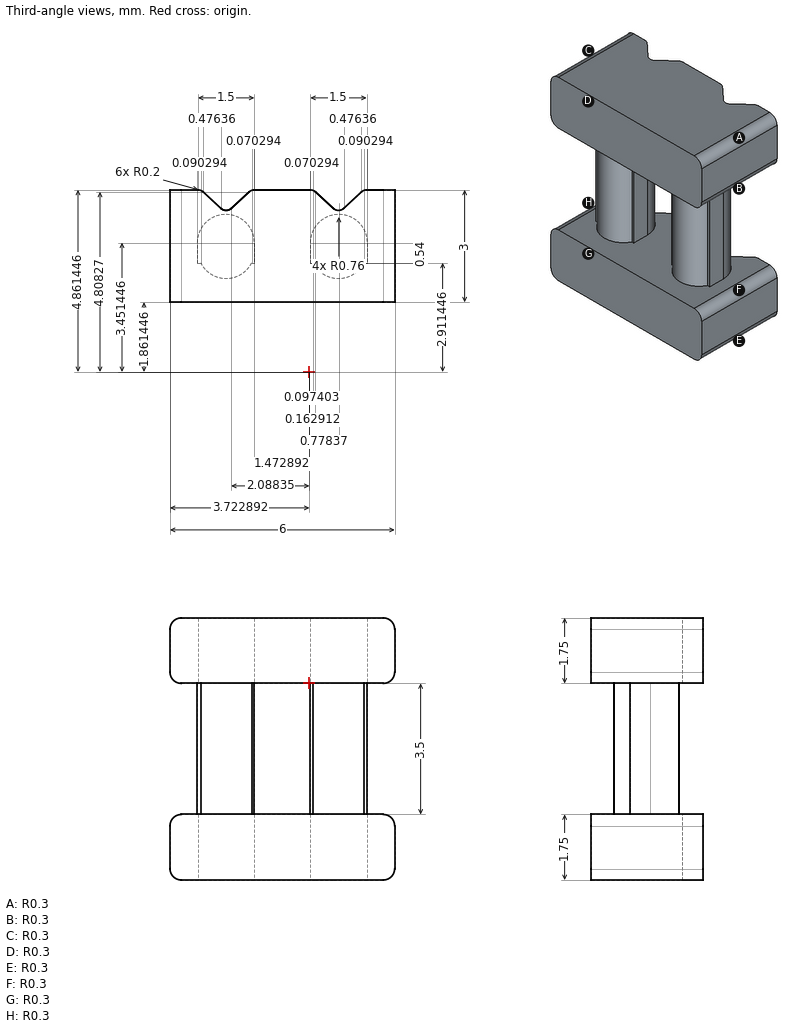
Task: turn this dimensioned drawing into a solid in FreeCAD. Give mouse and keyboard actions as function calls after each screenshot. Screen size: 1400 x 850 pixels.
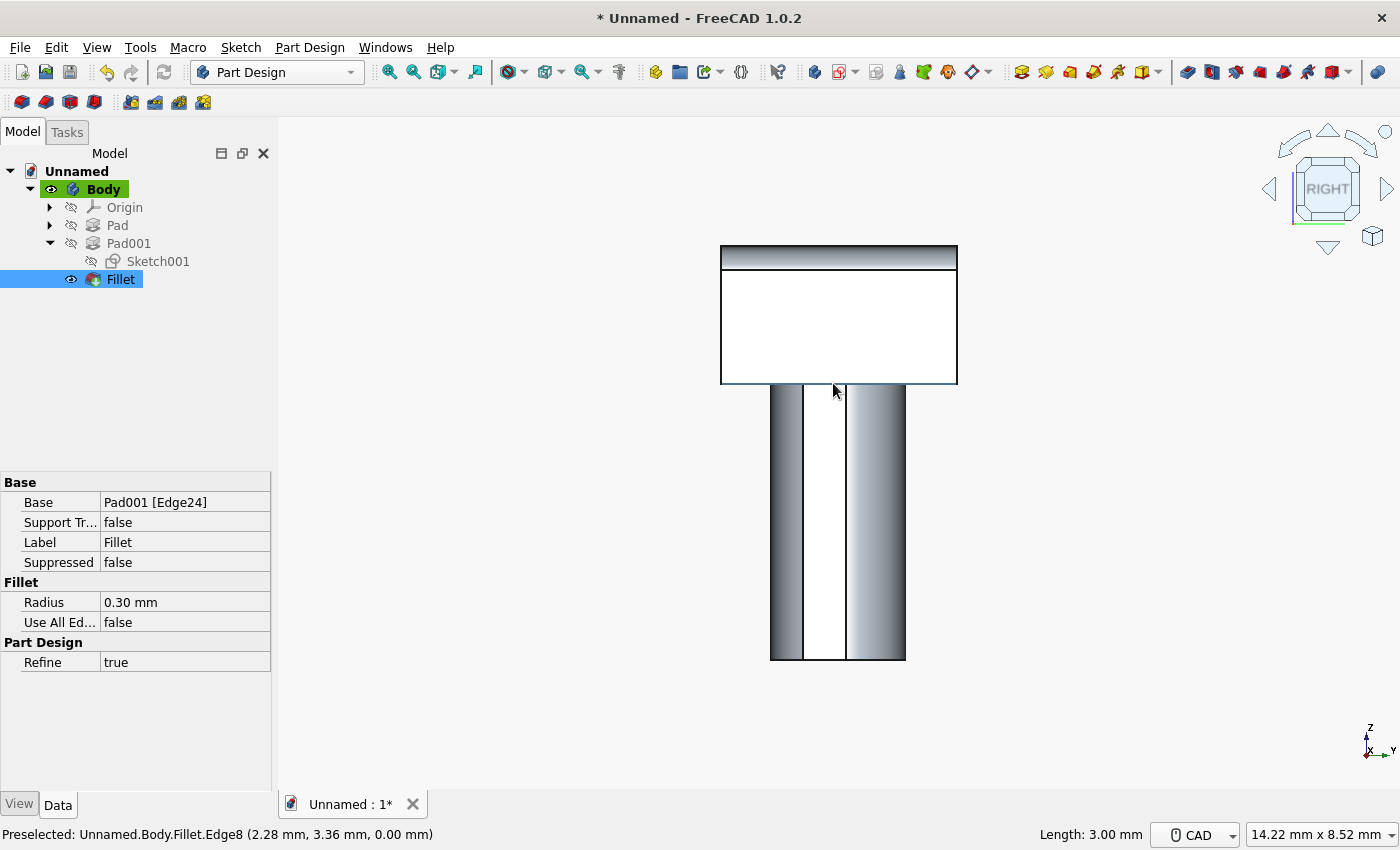
click(22, 102)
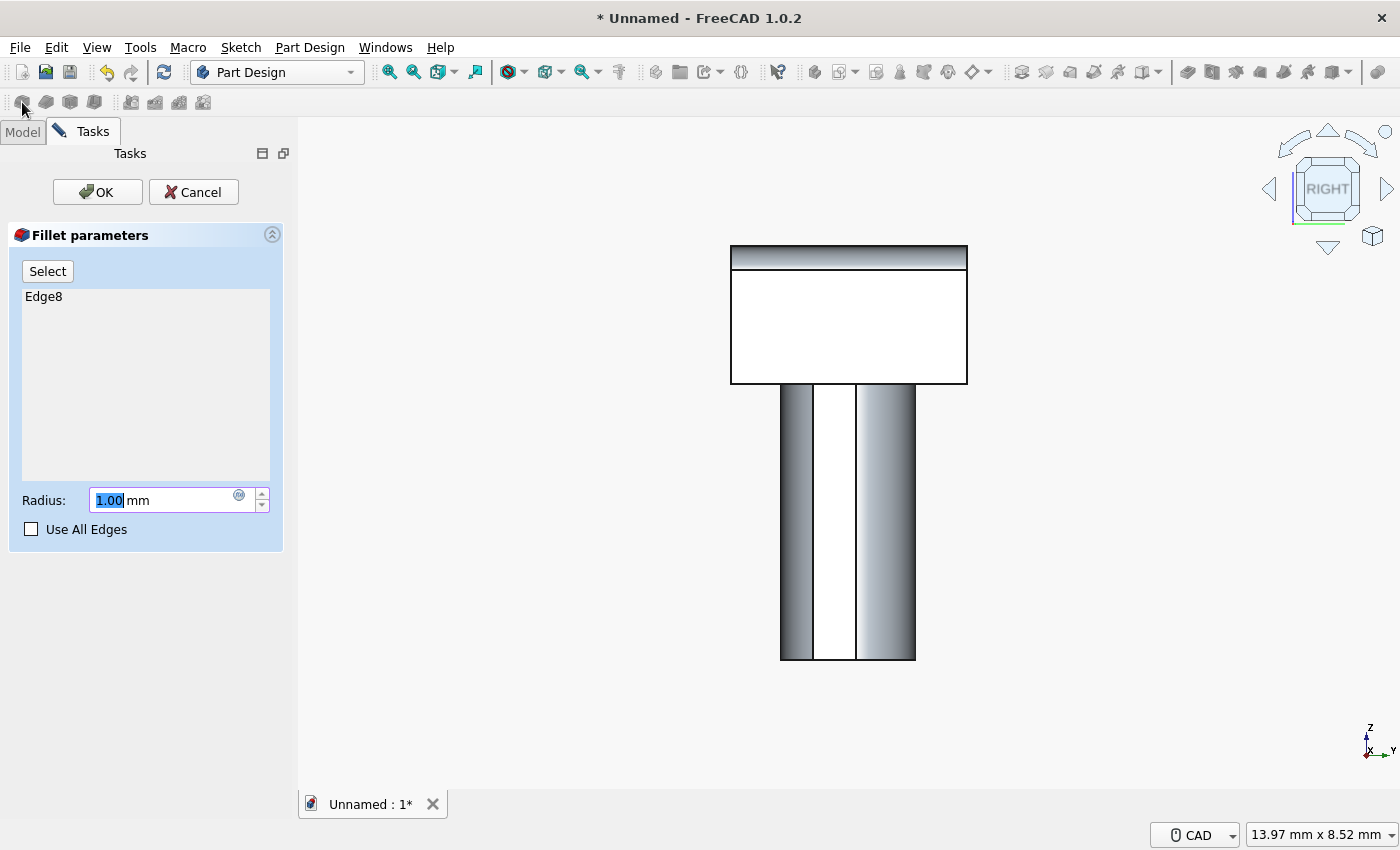
text(0.3)
key(Tab)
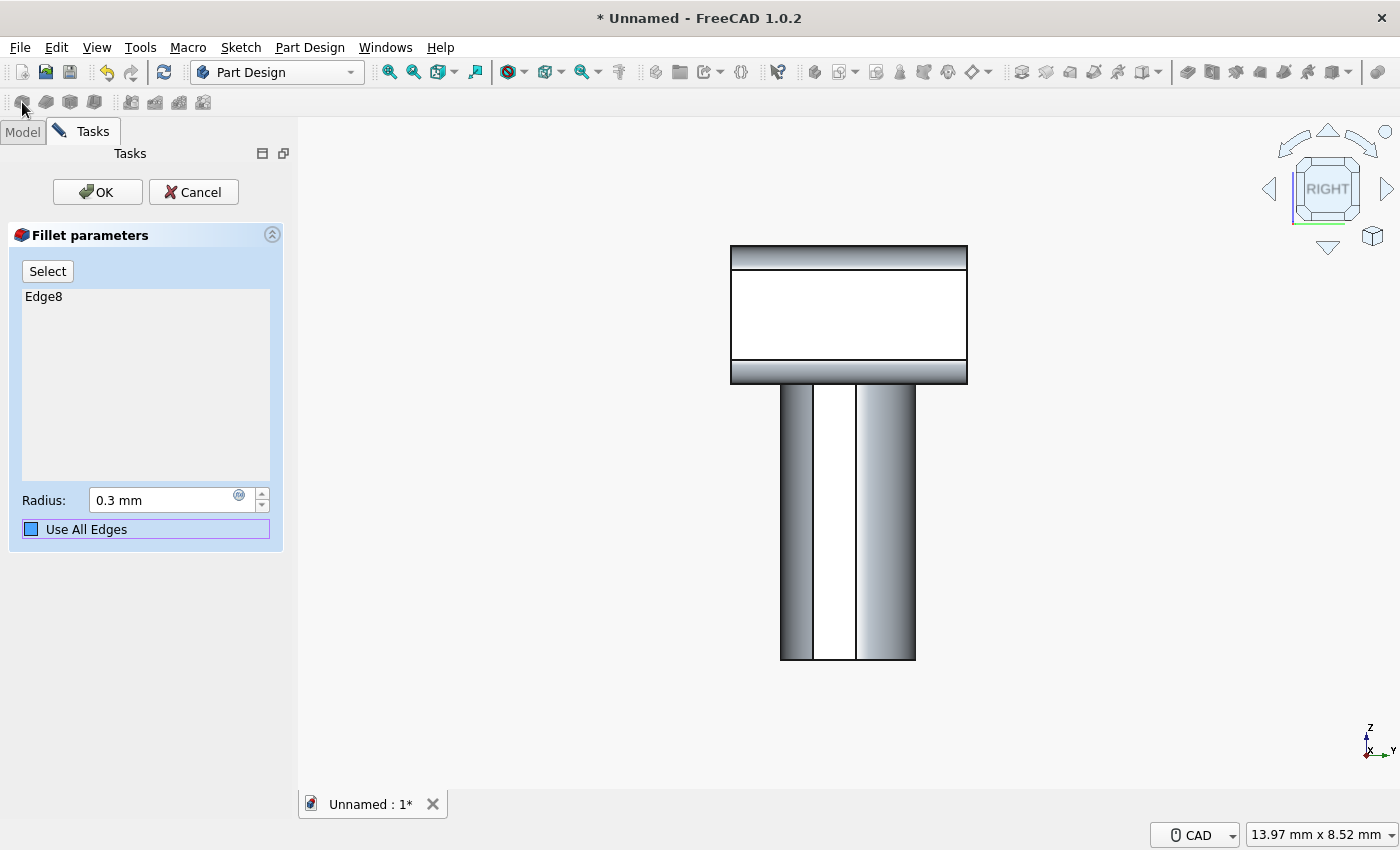
click(98, 192)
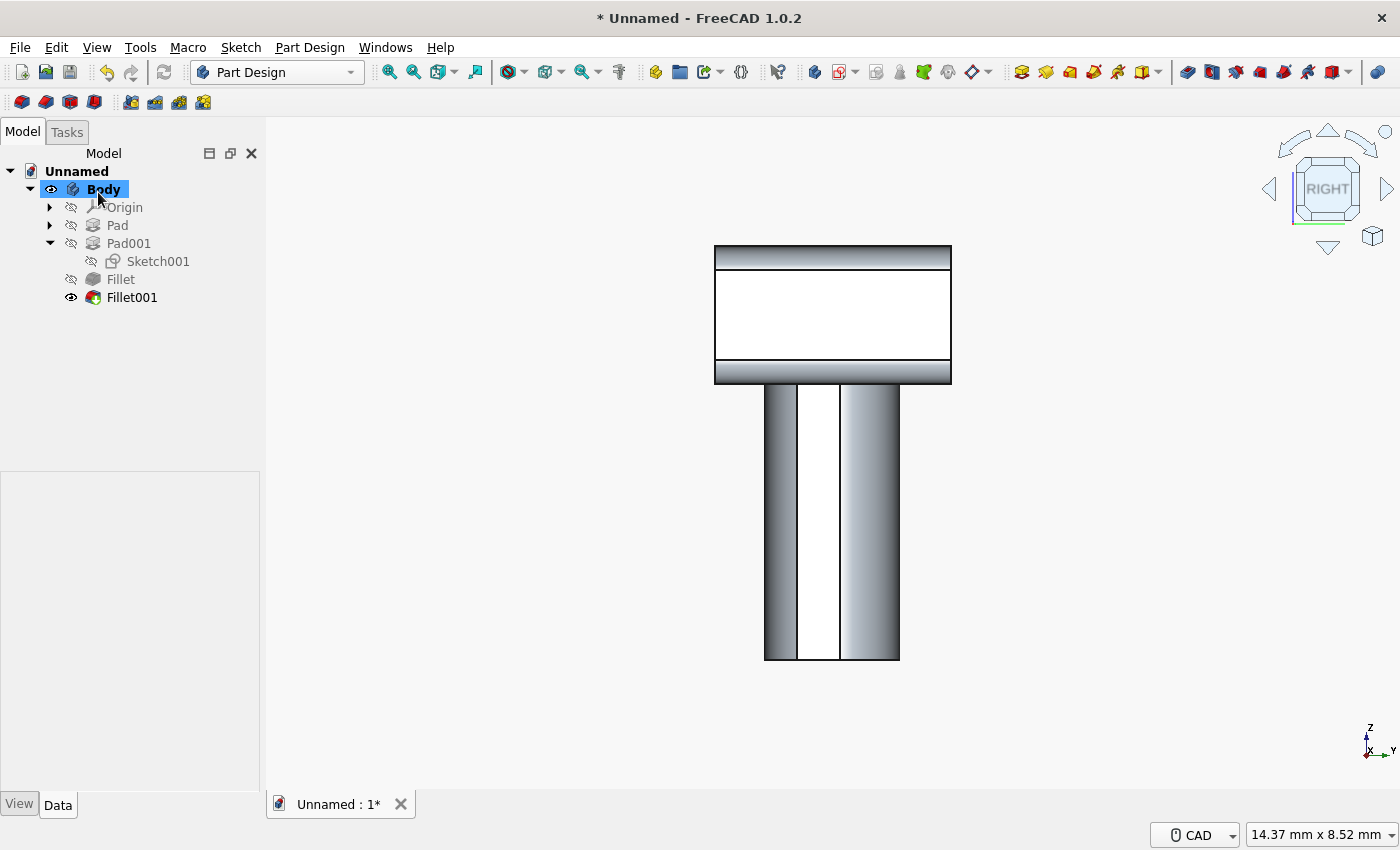
key(0)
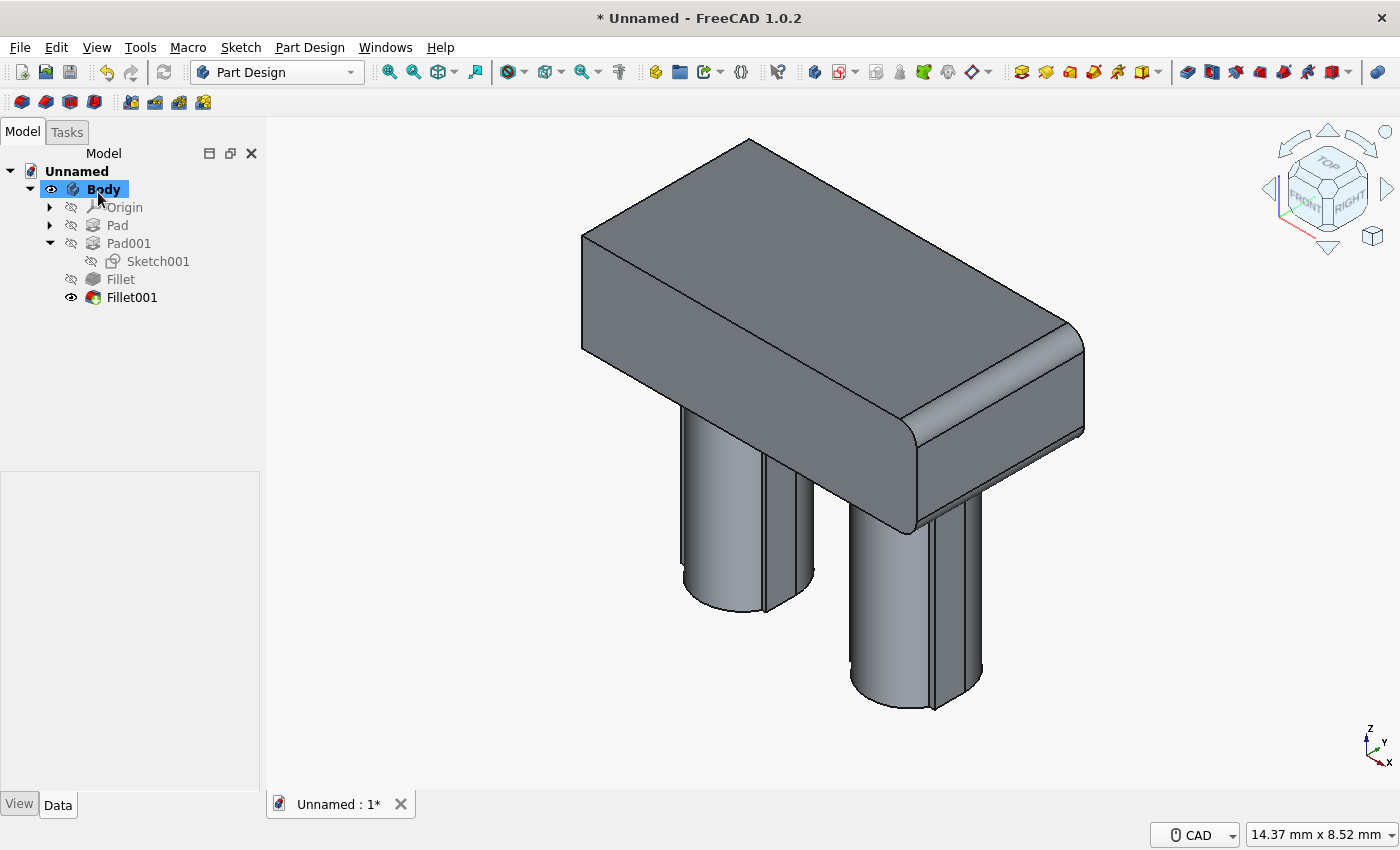
key(2)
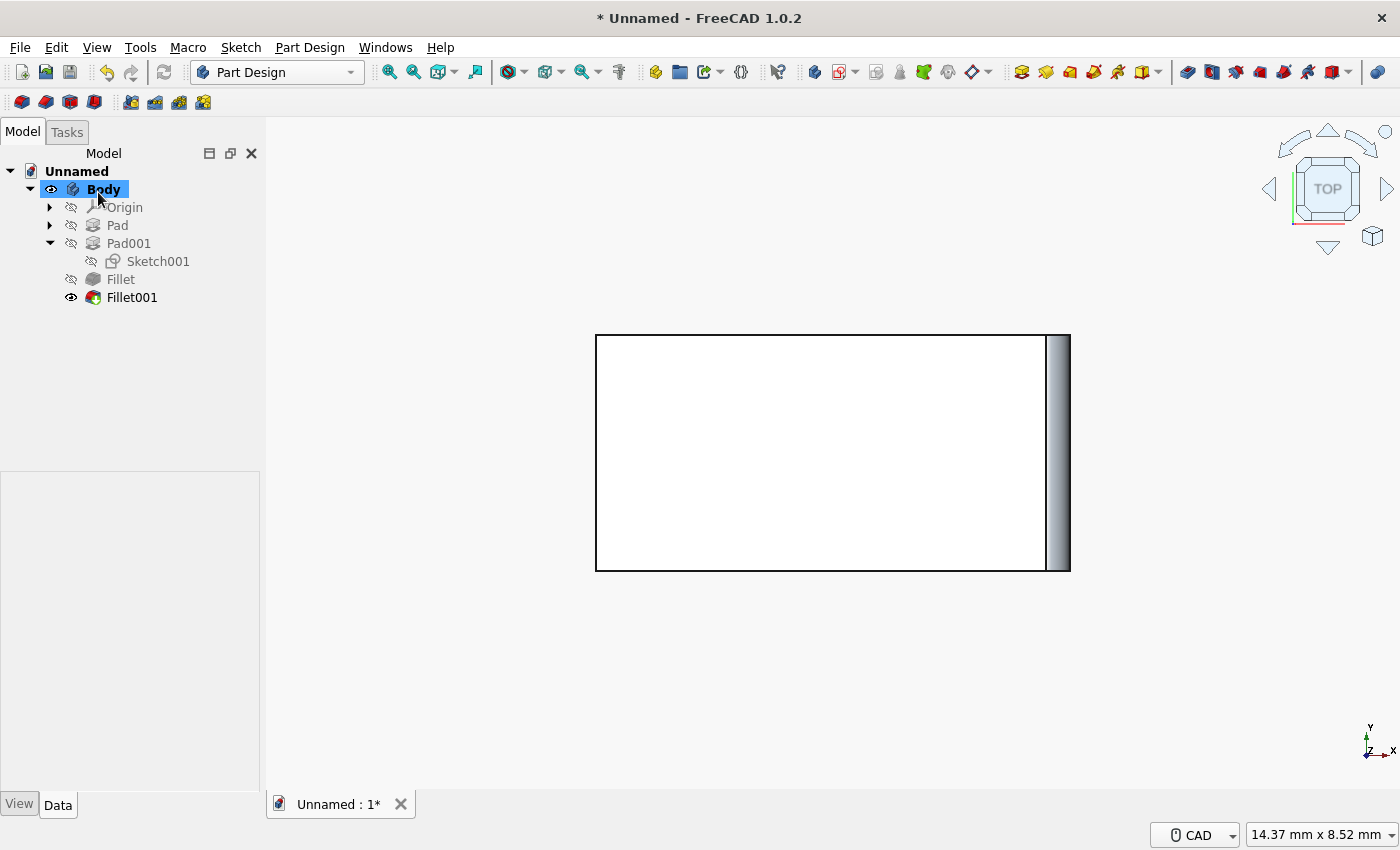
click(390, 72)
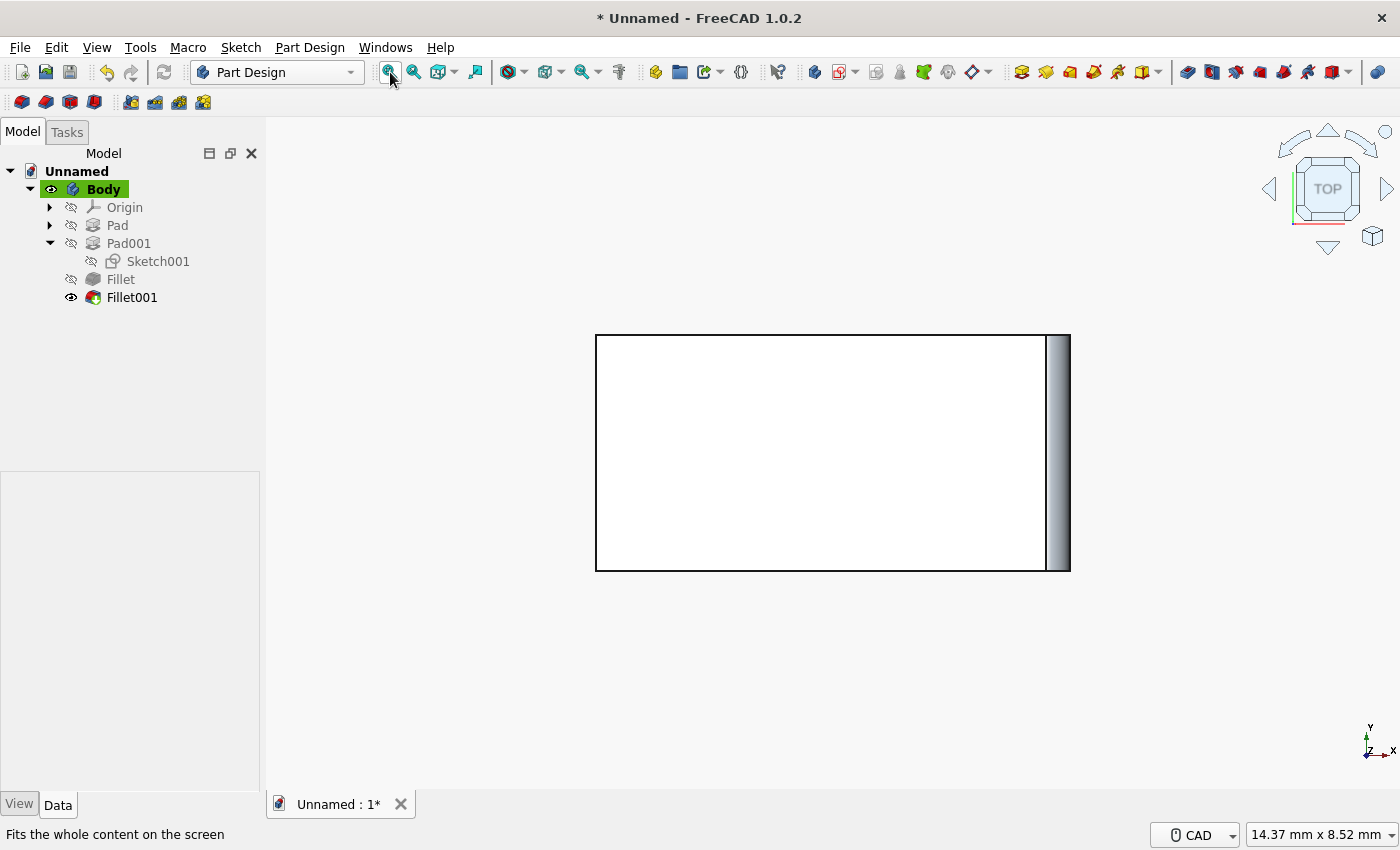
click(596, 452)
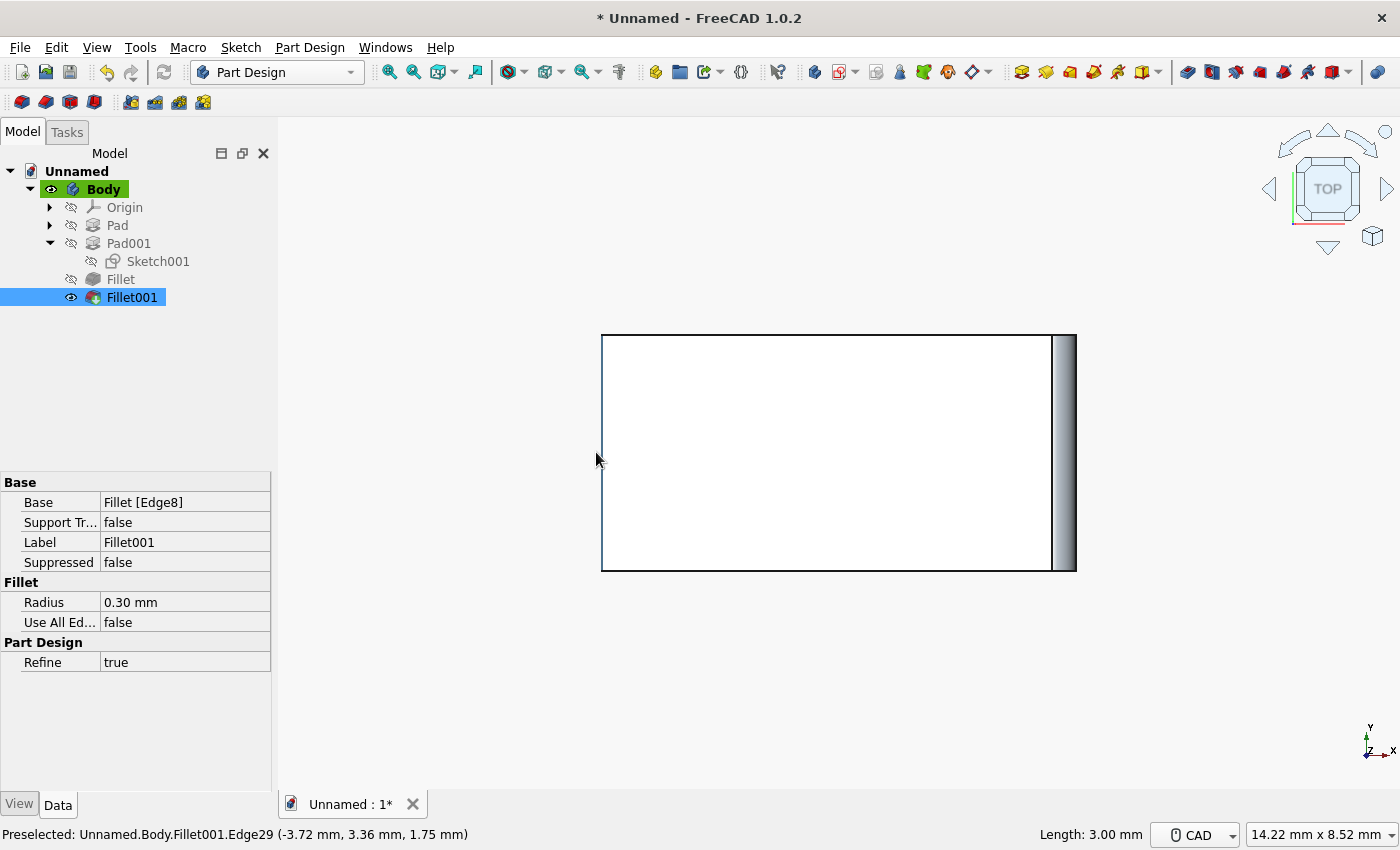
click(22, 102)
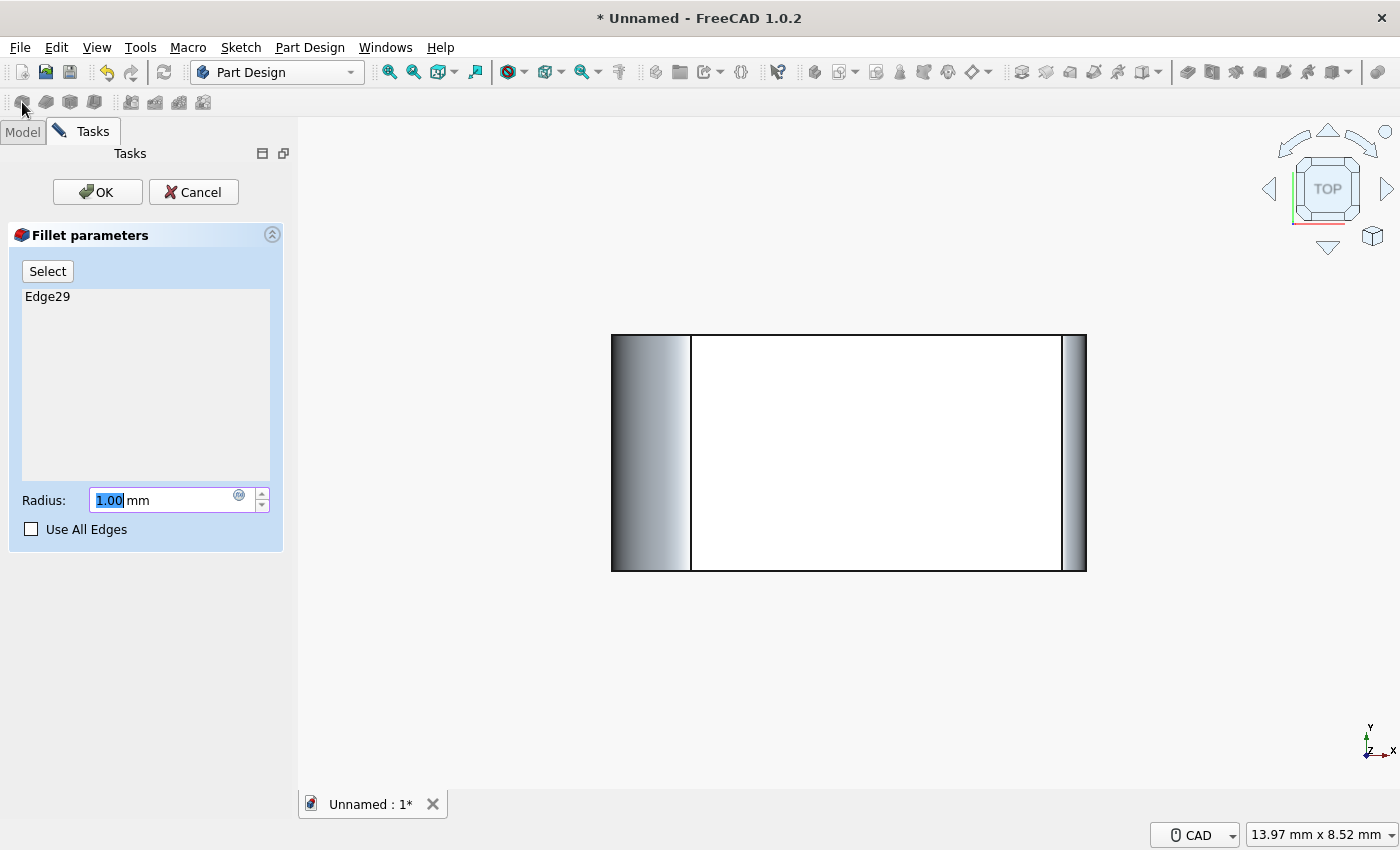
text(0.3)
key(Tab)